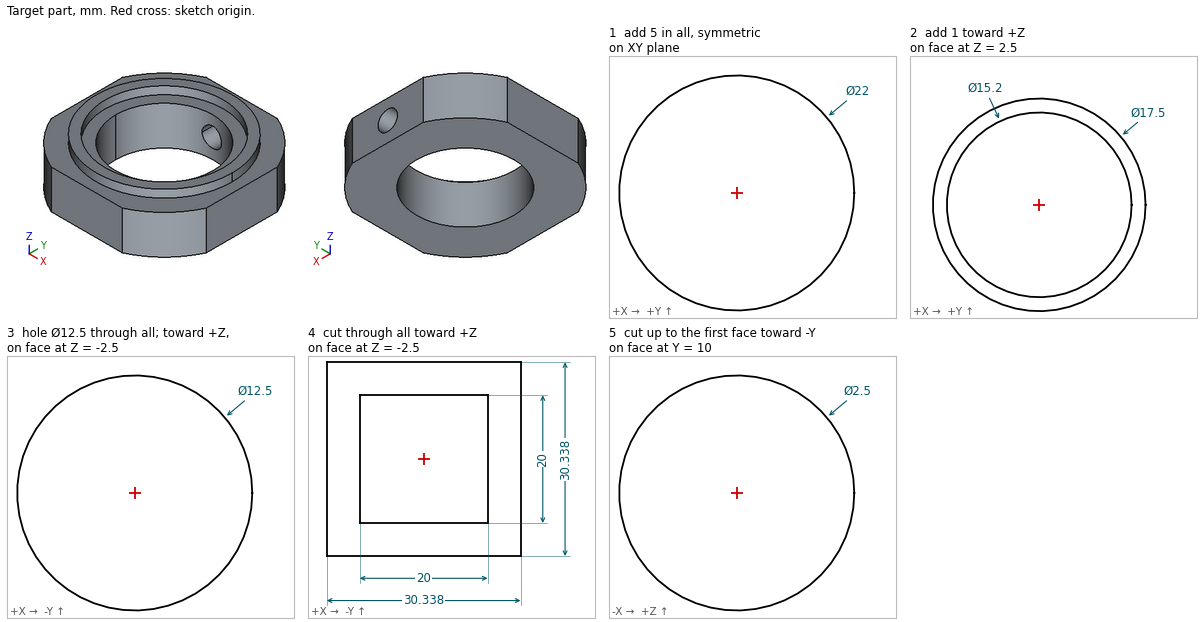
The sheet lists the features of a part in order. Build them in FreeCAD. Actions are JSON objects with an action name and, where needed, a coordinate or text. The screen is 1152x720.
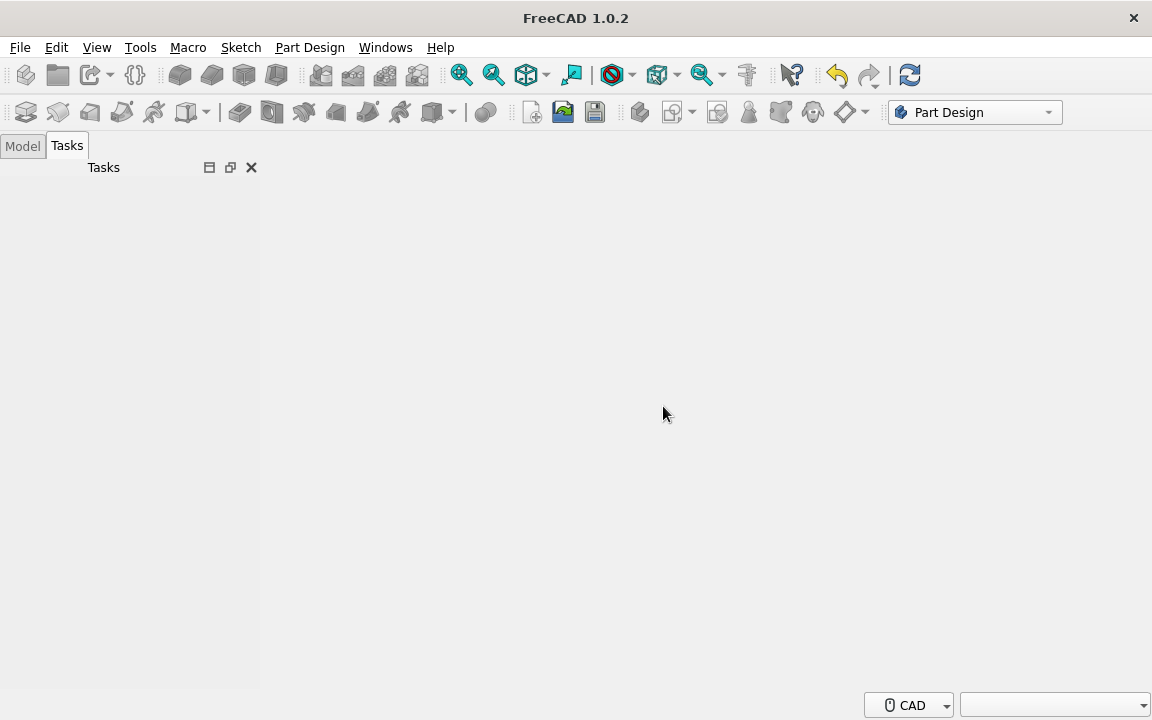
{"action": "left_click", "coordinate": [532, 112]}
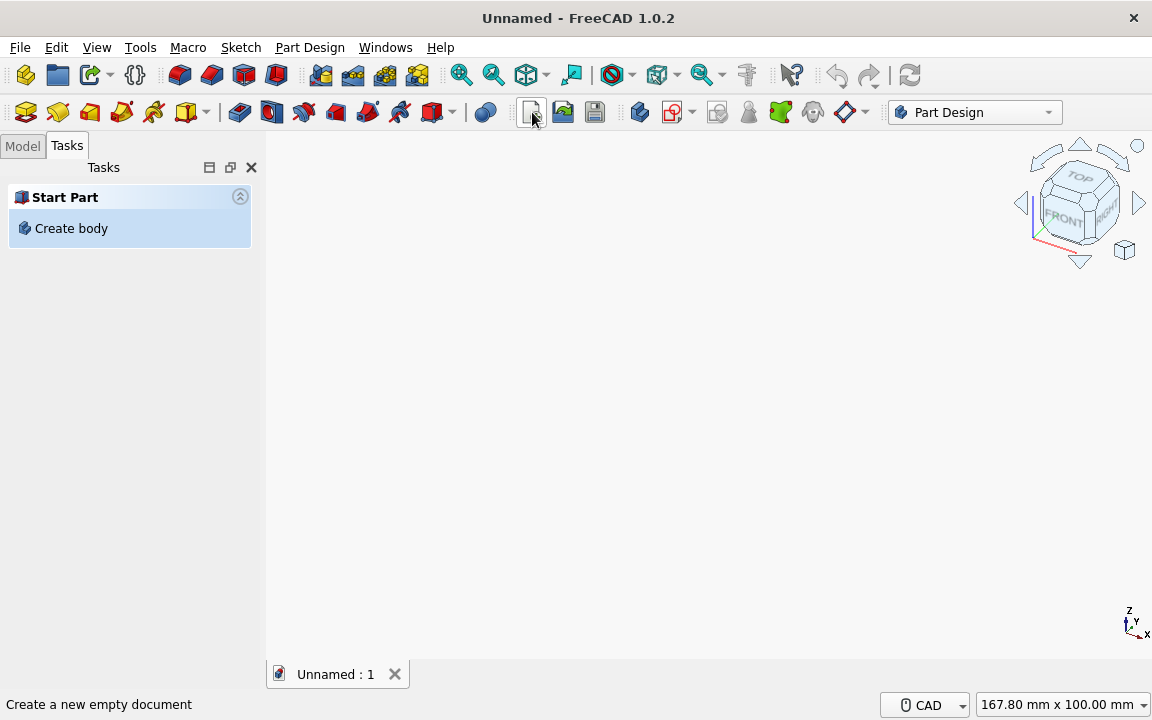
{"action": "left_click", "coordinate": [672, 112]}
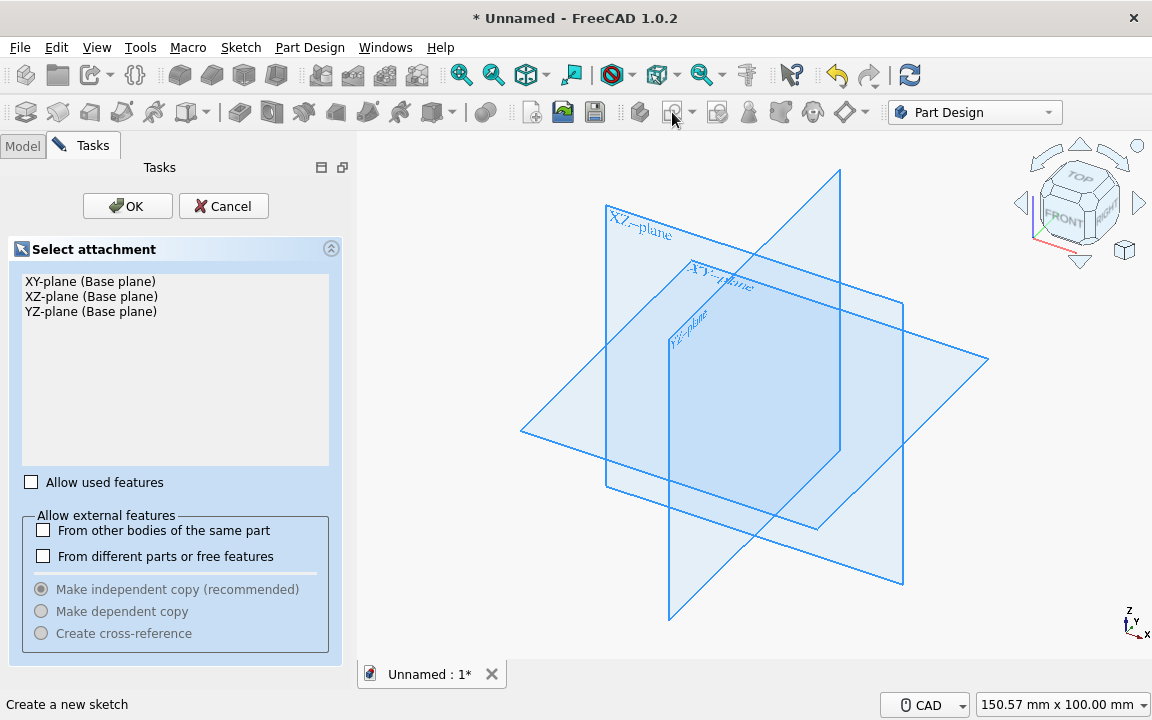
{"action": "left_click", "coordinate": [82, 282]}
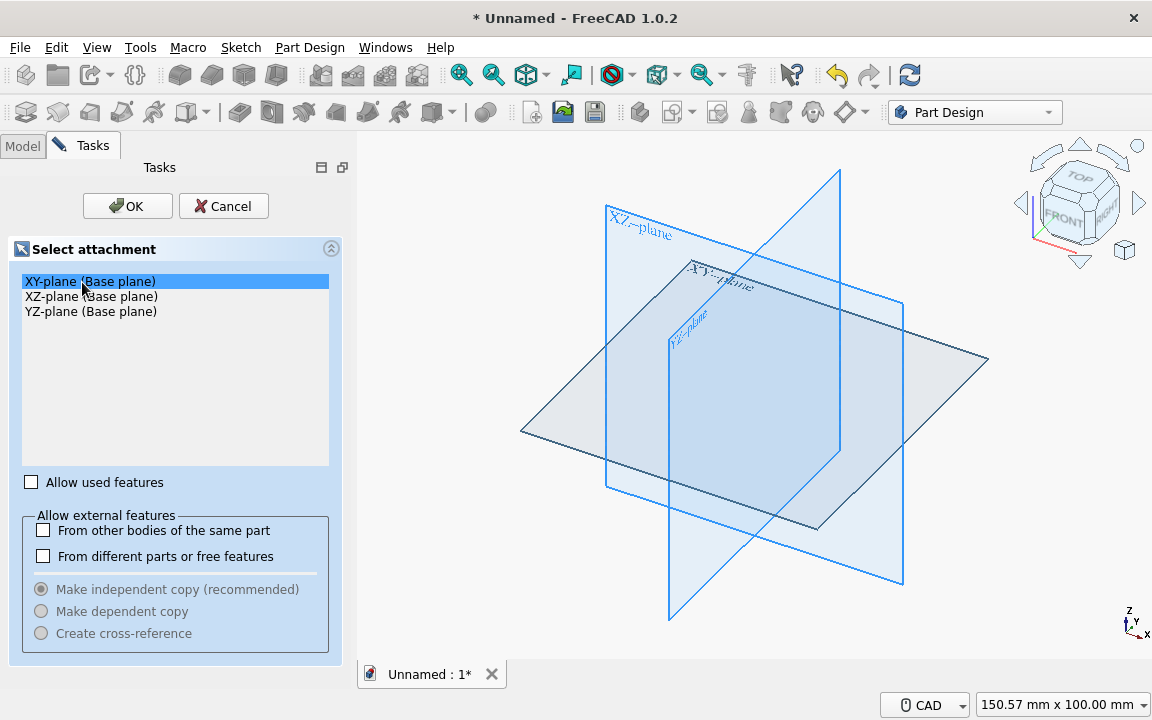
{"action": "left_click", "coordinate": [128, 206]}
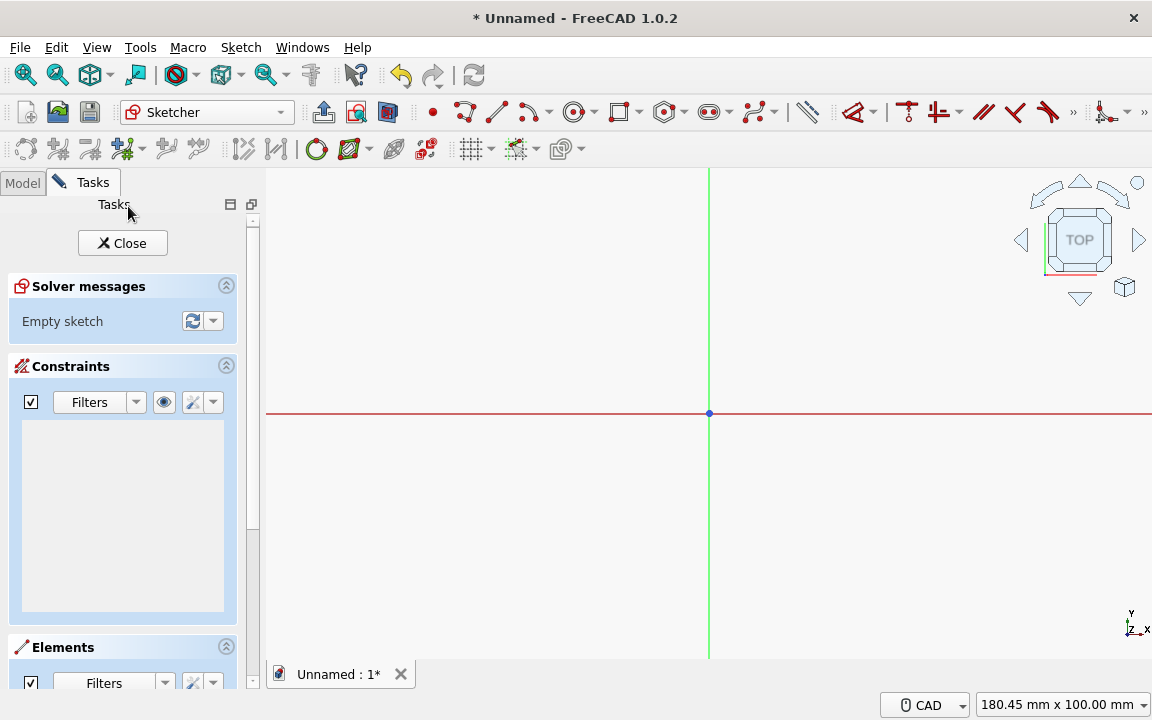
{"action": "scroll", "coordinate": [749, 414], "scroll_direction": "up", "scroll_amount": 5}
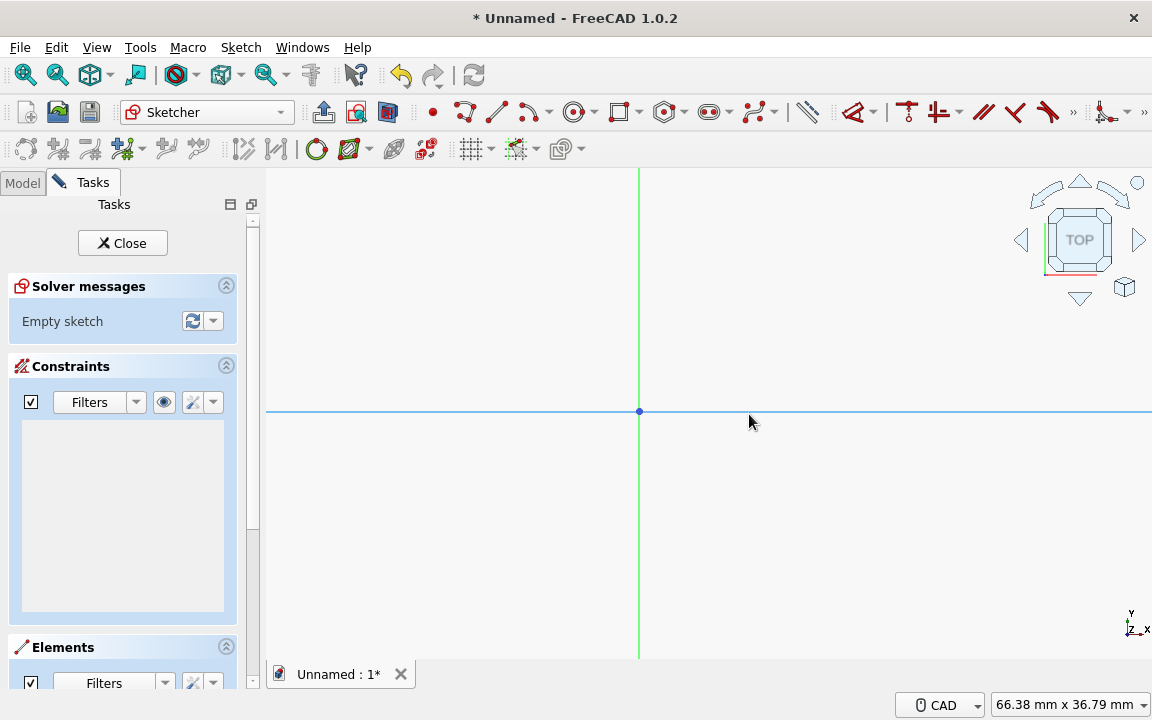
{"action": "left_click", "coordinate": [574, 112]}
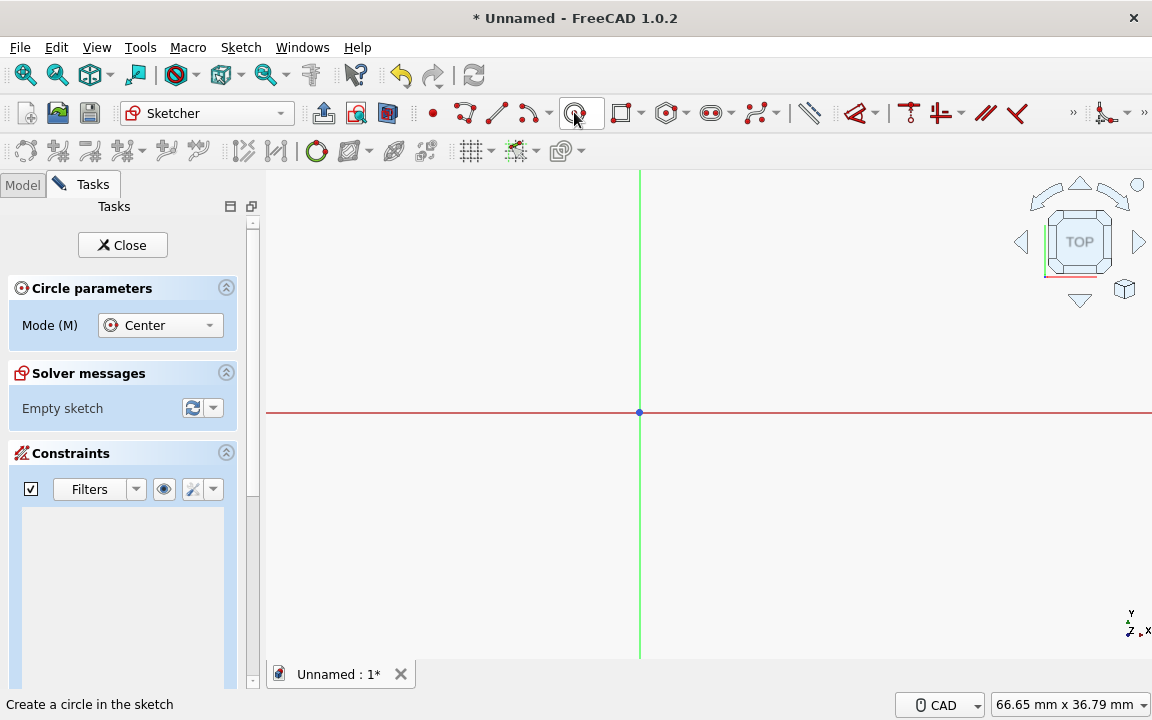
{"action": "left_click", "coordinate": [640, 413]}
{"action": "mouse_move", "coordinate": [743, 309]}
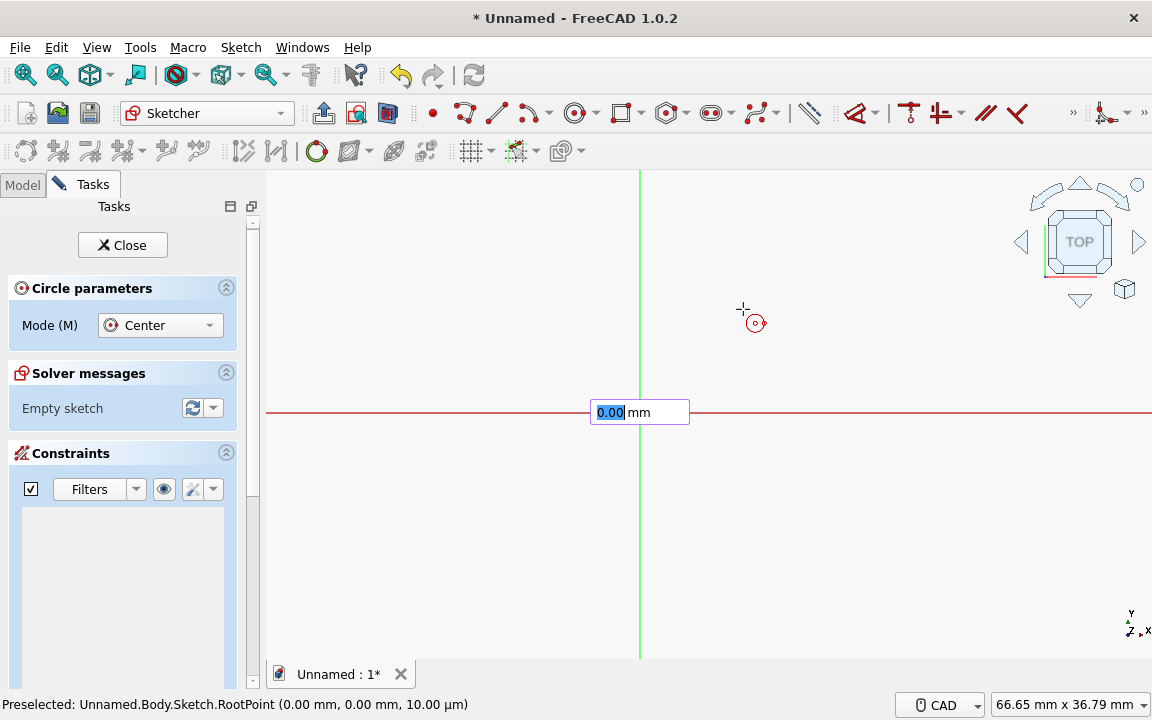
{"action": "type", "text": "22"}
{"action": "key", "text": "Return"}
{"action": "key", "text": "Escape"}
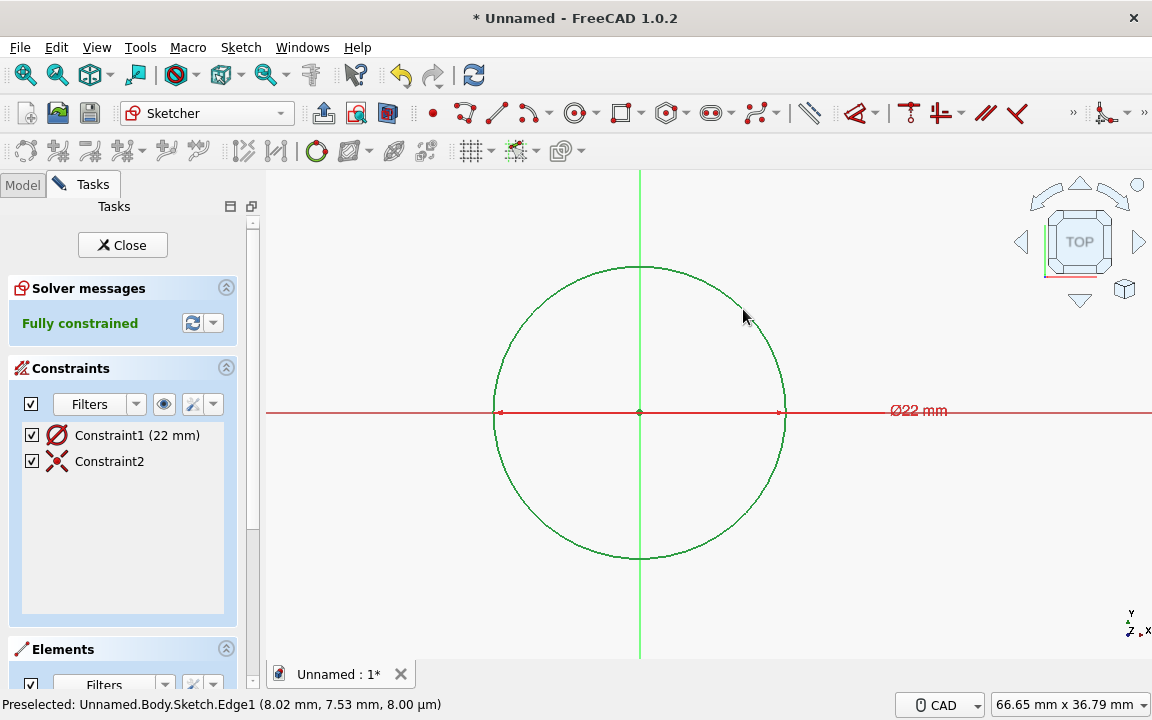
{"action": "left_click", "coordinate": [123, 245]}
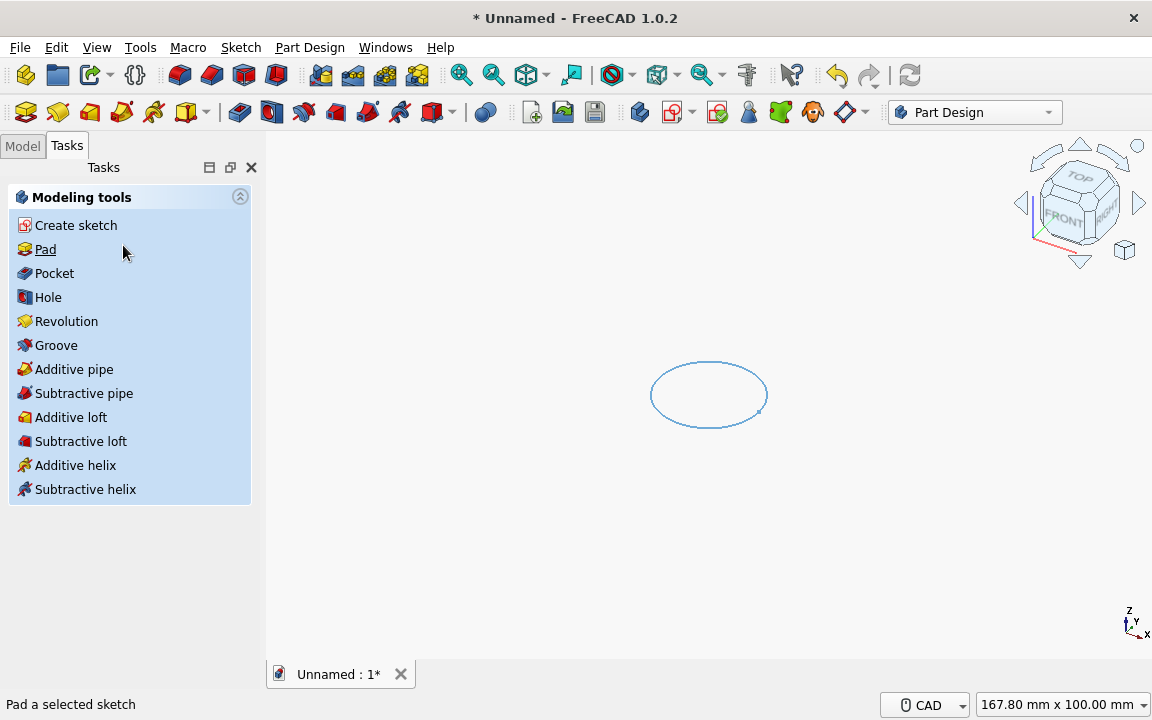
{"action": "left_click", "coordinate": [26, 112]}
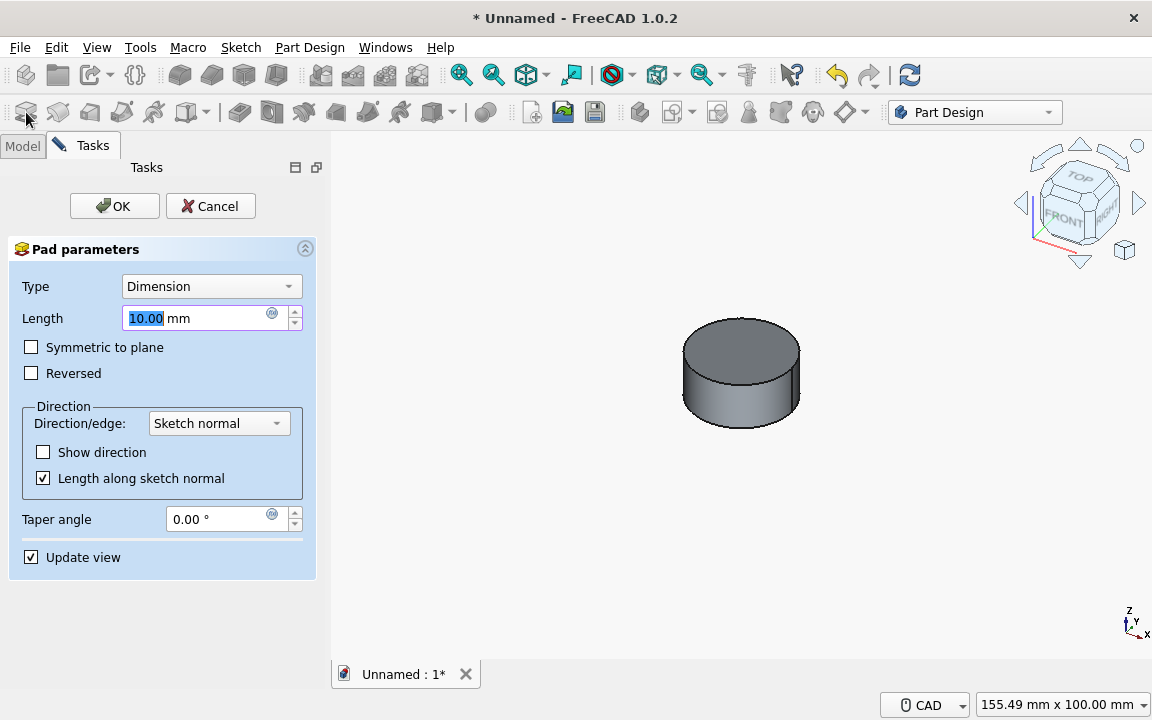
{"action": "type", "text": "5"}
{"action": "key", "text": "Tab"}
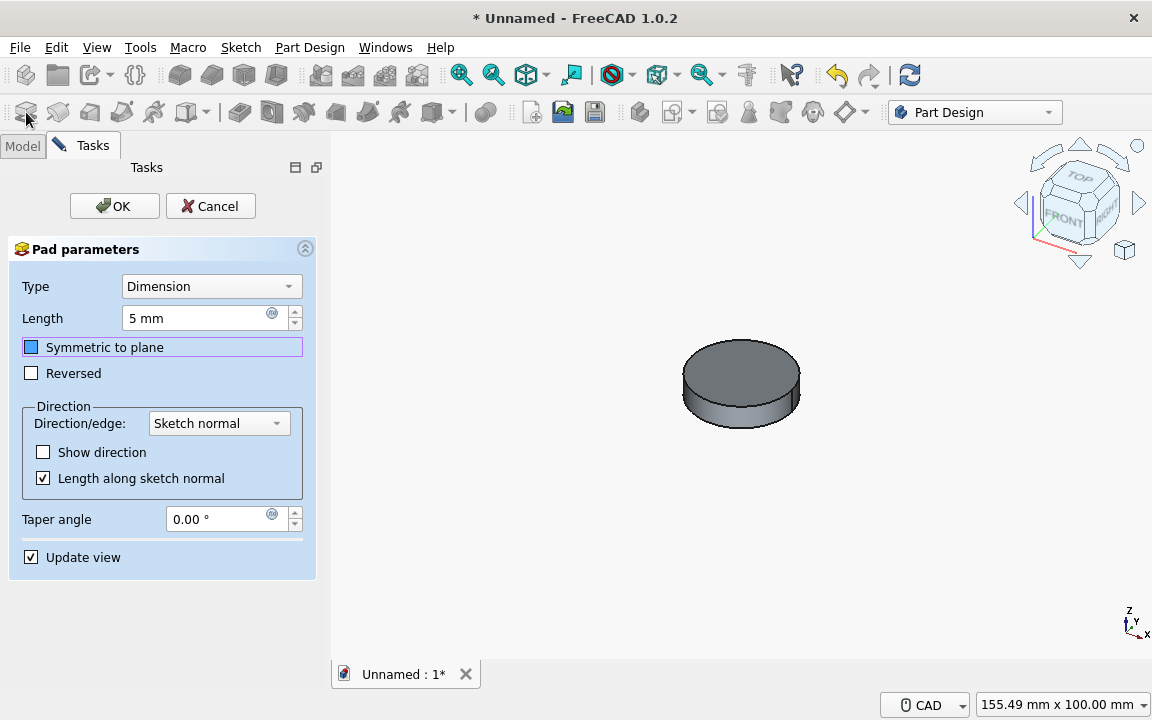
{"action": "left_click", "coordinate": [30, 347]}